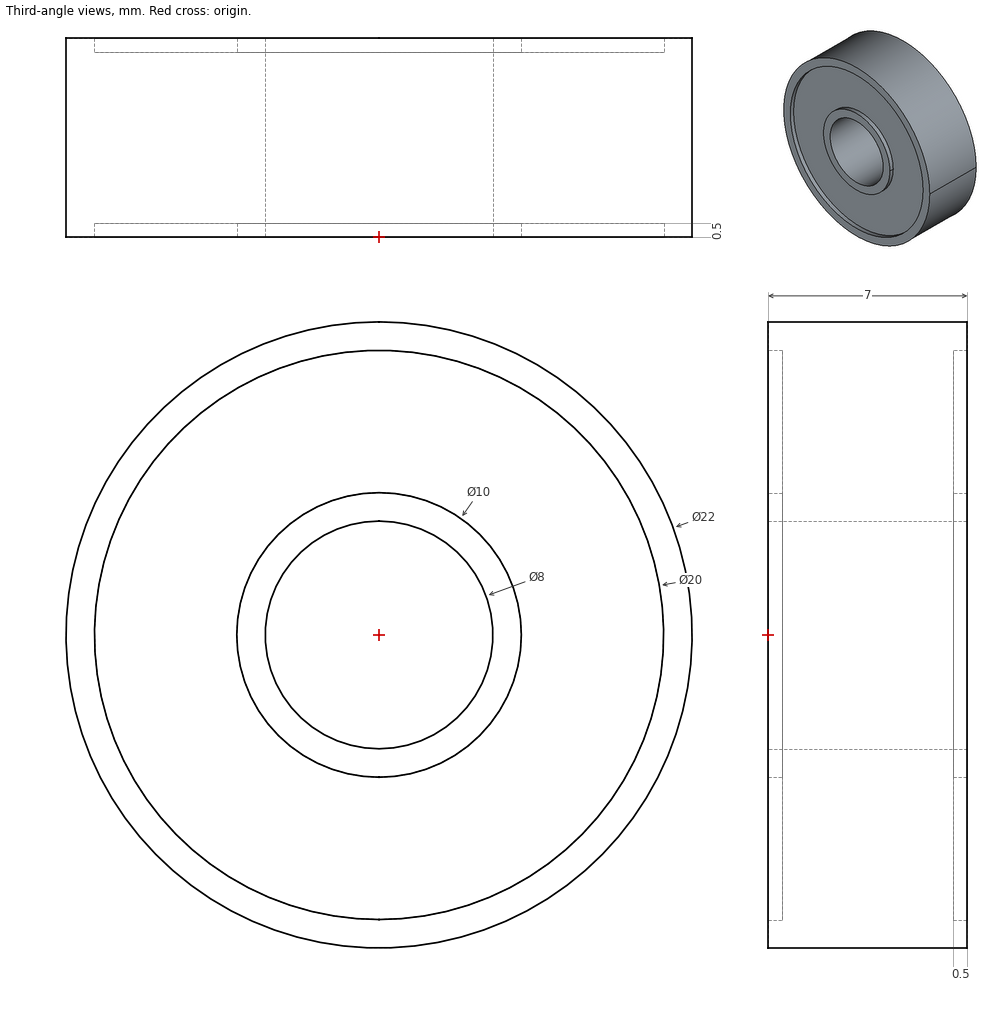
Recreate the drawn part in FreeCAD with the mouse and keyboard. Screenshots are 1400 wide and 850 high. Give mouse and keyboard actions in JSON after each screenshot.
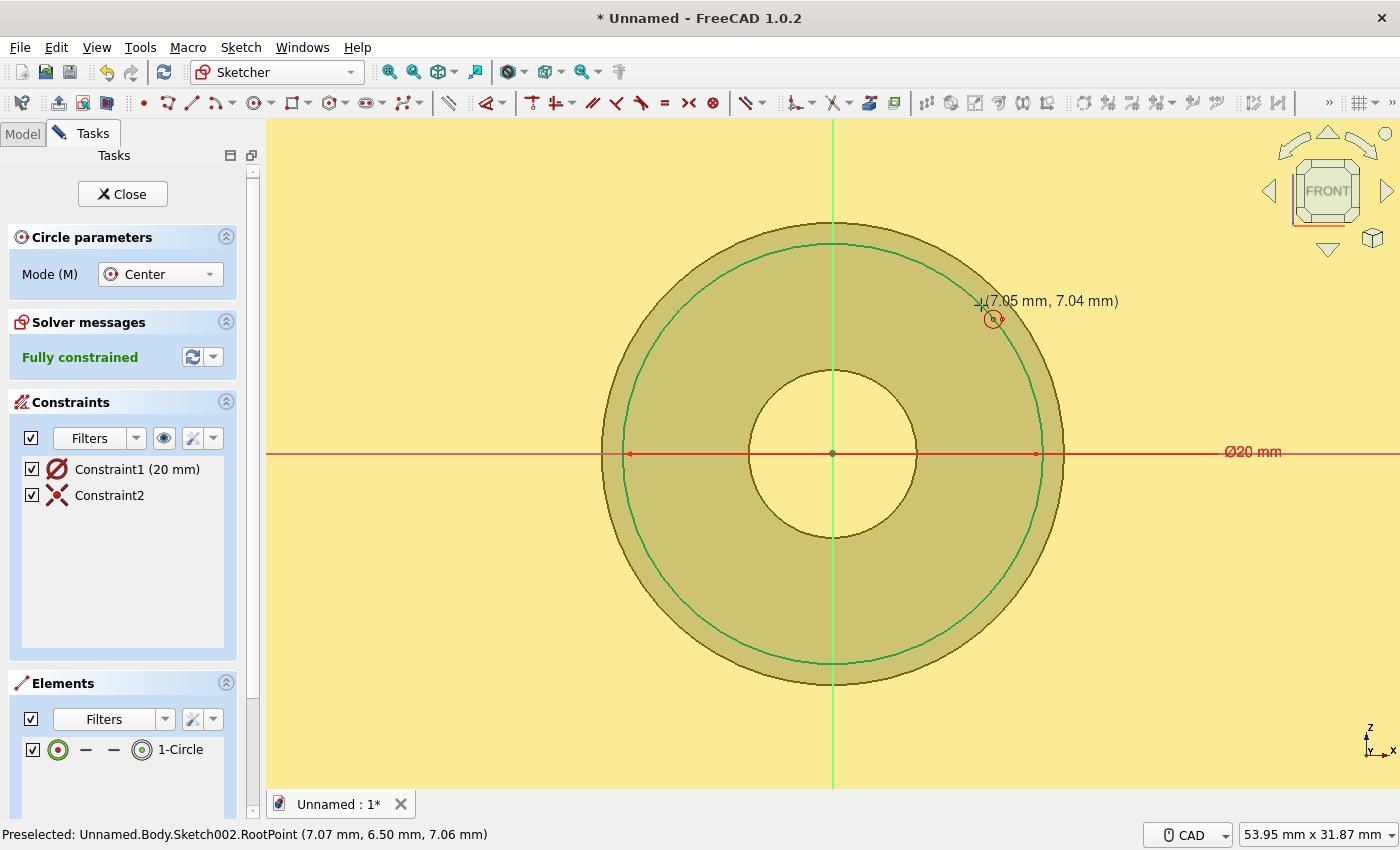
{"action": "left_click", "coordinate": [833, 454]}
{"action": "mouse_move", "coordinate": [907, 380]}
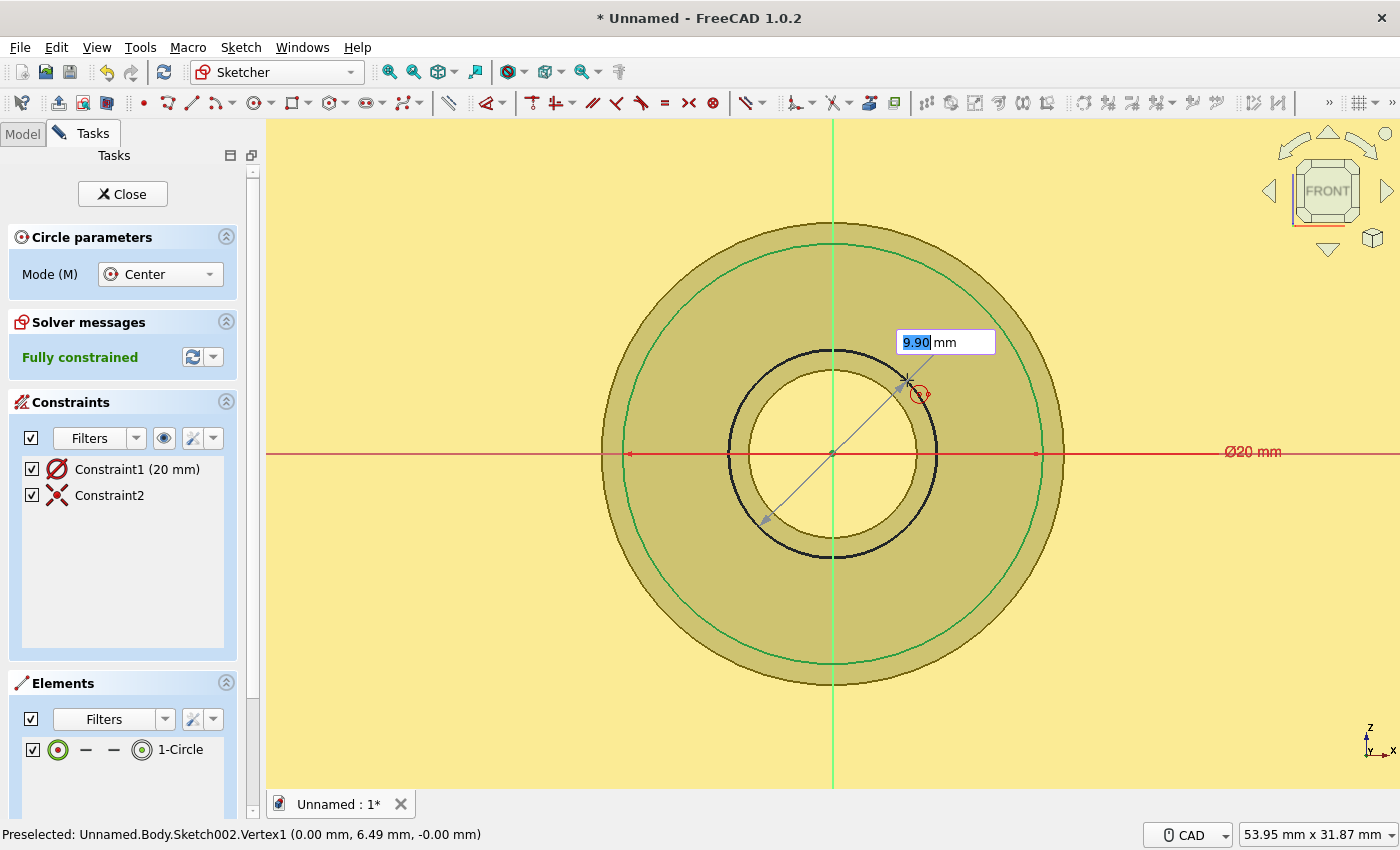
{"action": "type", "text": "10"}
{"action": "key", "text": "Return"}
{"action": "key", "text": "Escape"}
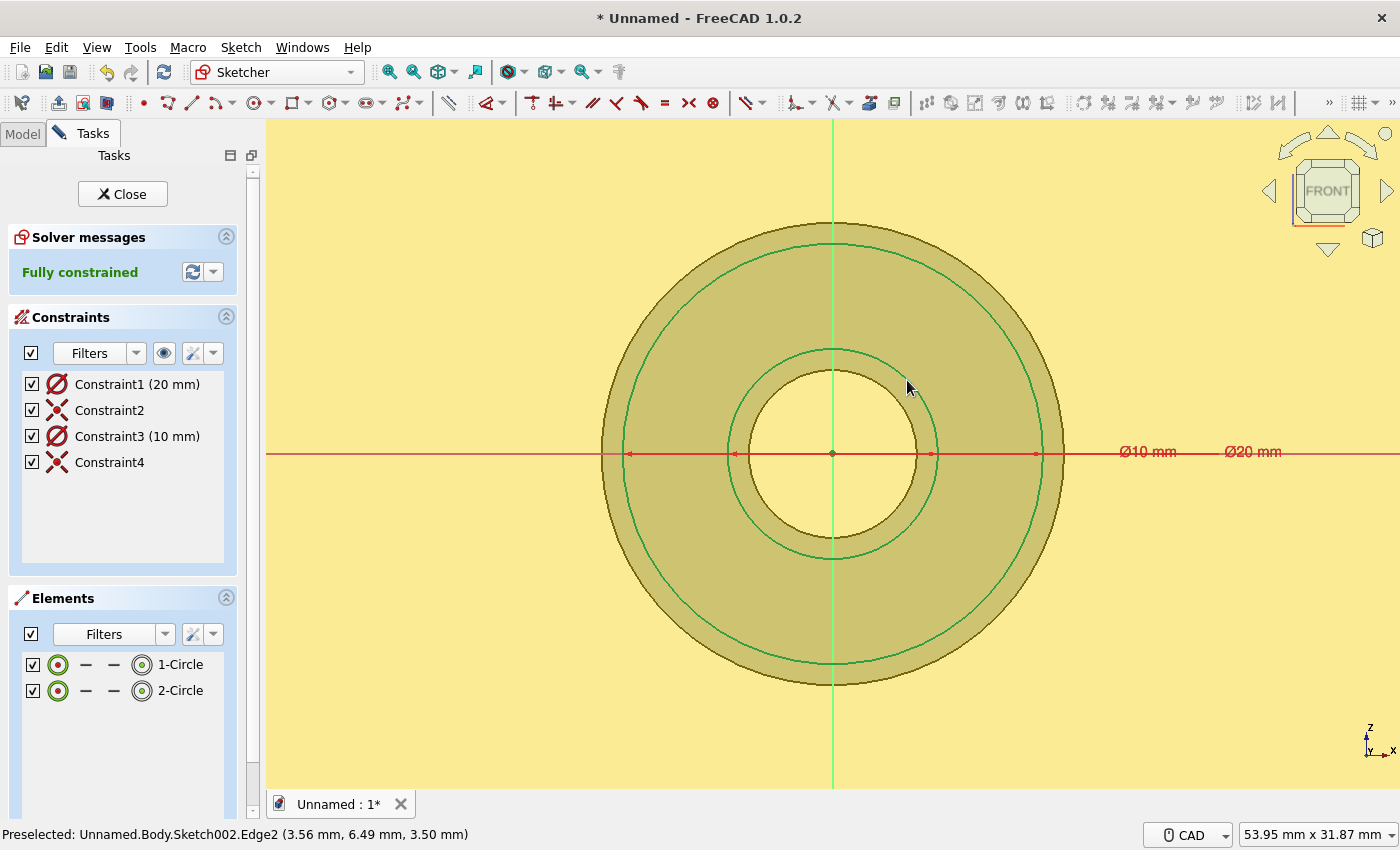
{"action": "left_click", "coordinate": [123, 194]}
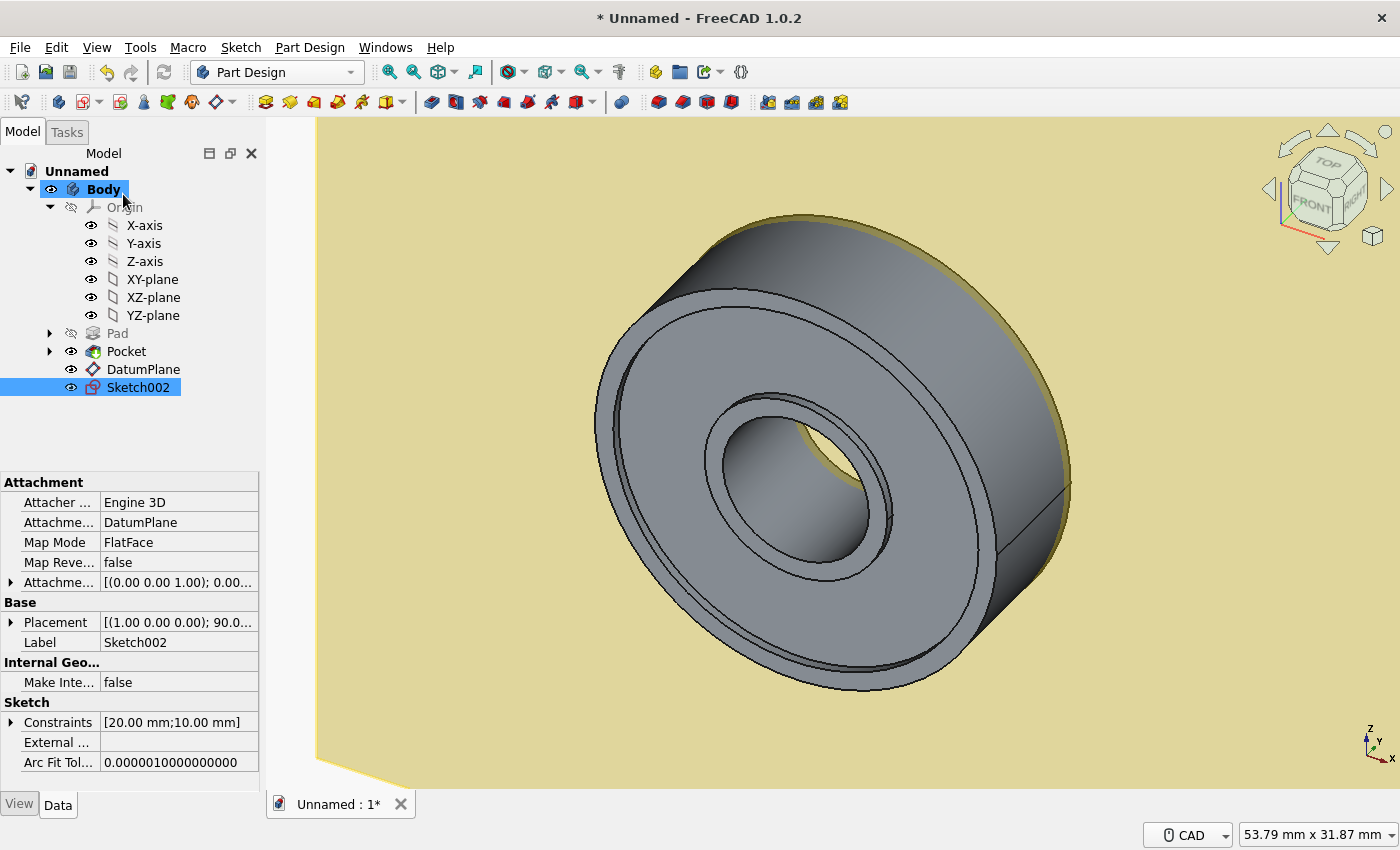
{"action": "left_click", "coordinate": [432, 102]}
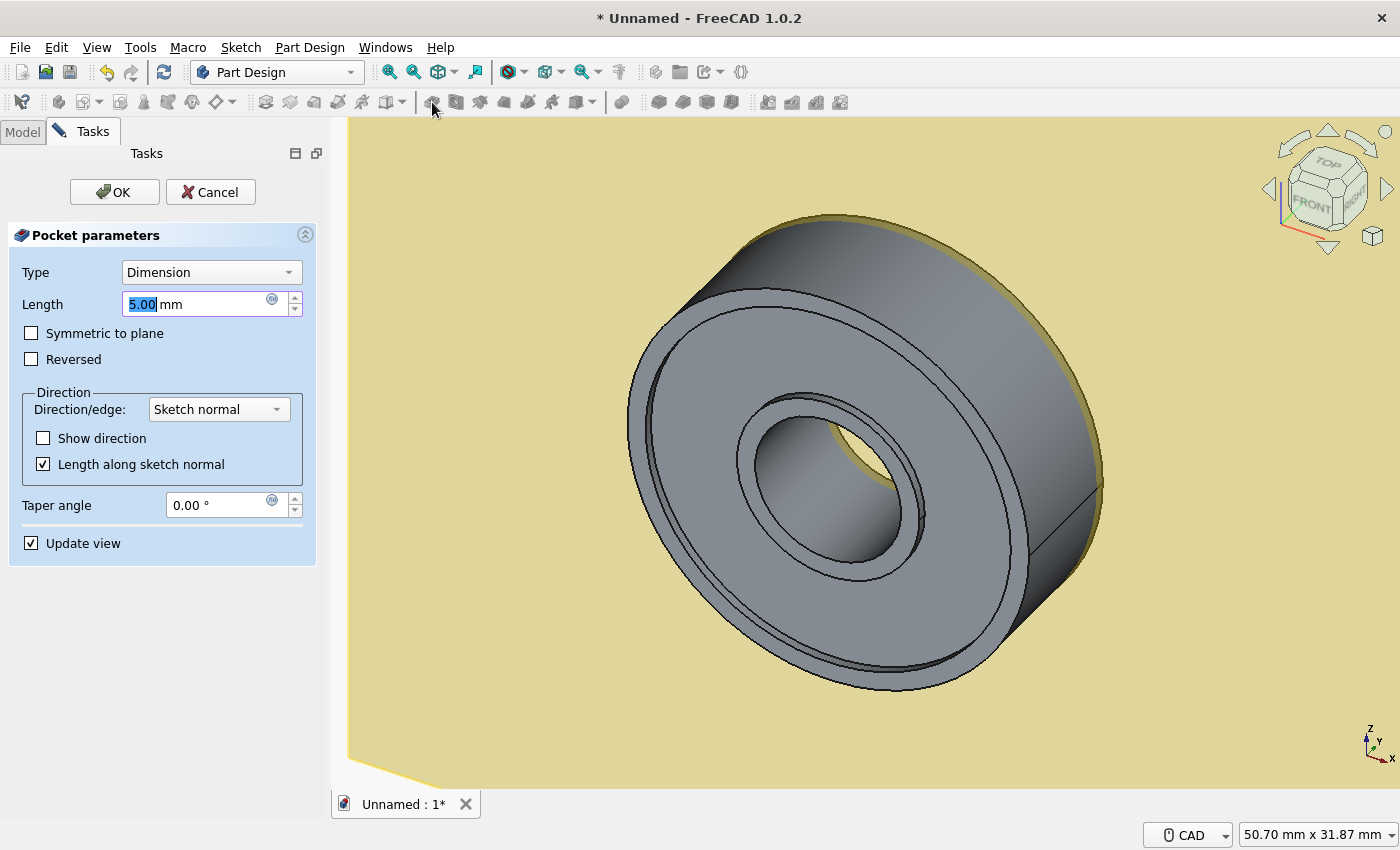
{"action": "type", "text": "0.5"}
{"action": "key", "text": "Tab"}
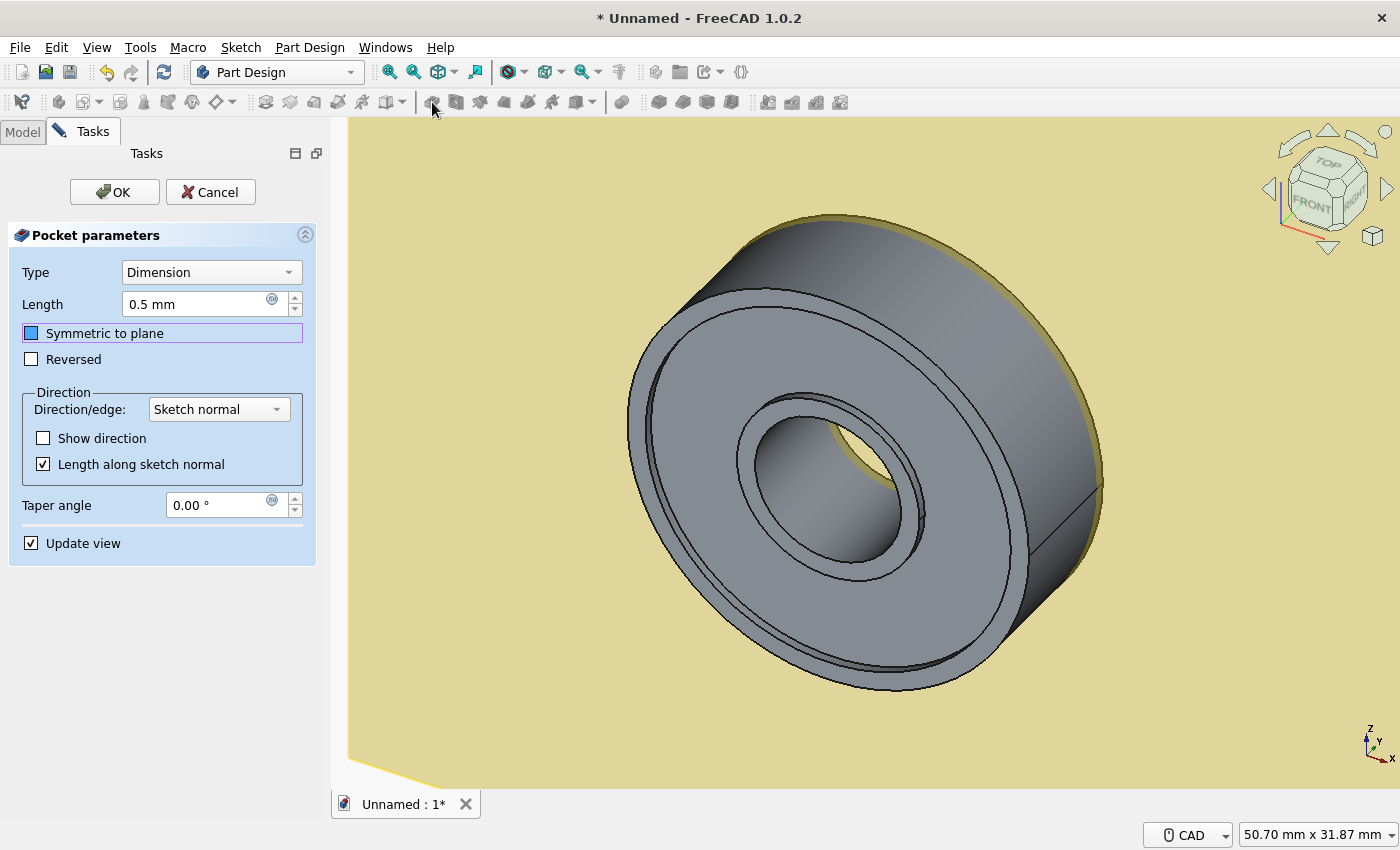
{"action": "left_click", "coordinate": [115, 192]}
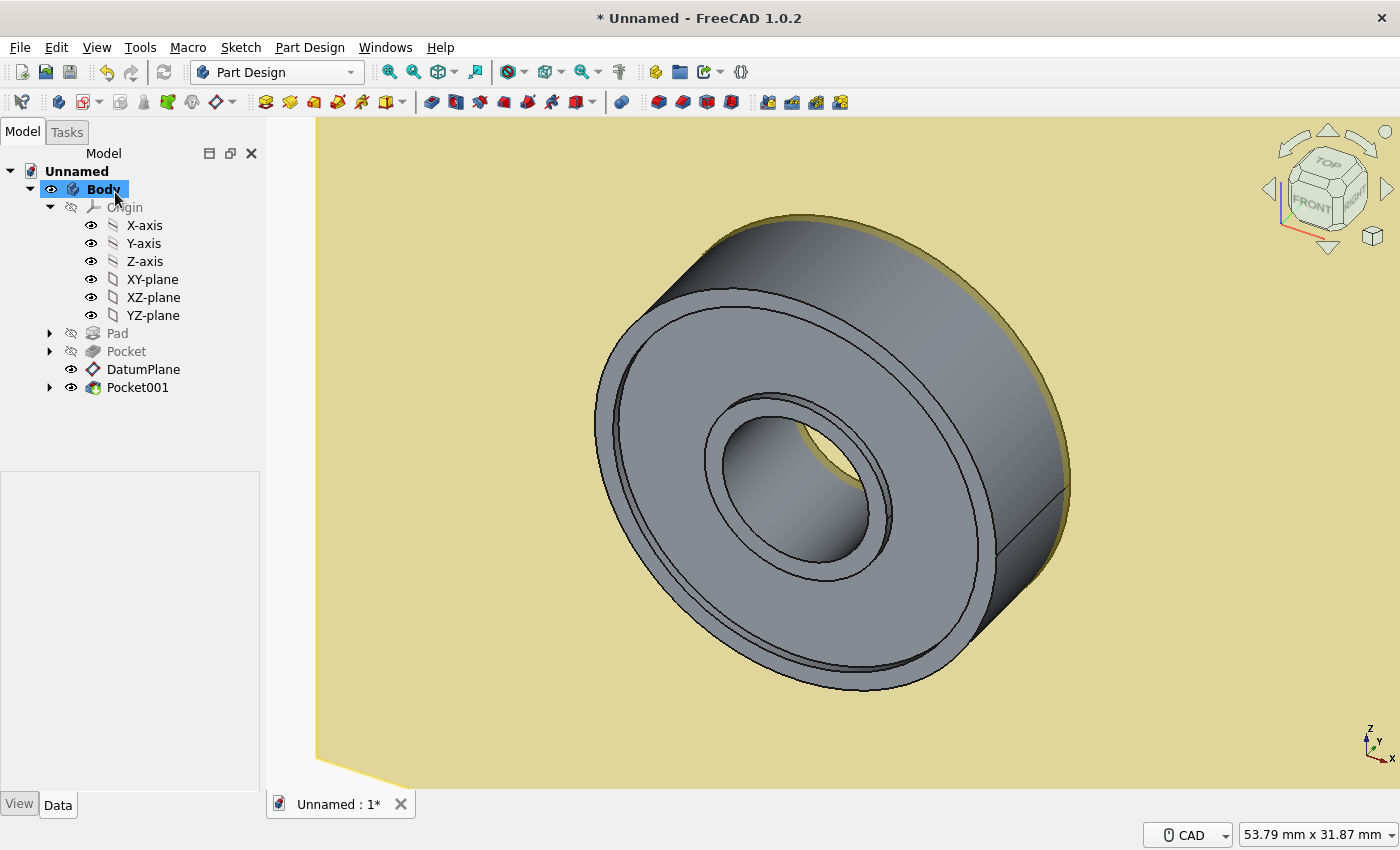
{"action": "left_click", "coordinate": [116, 369]}
{"action": "key", "text": "space"}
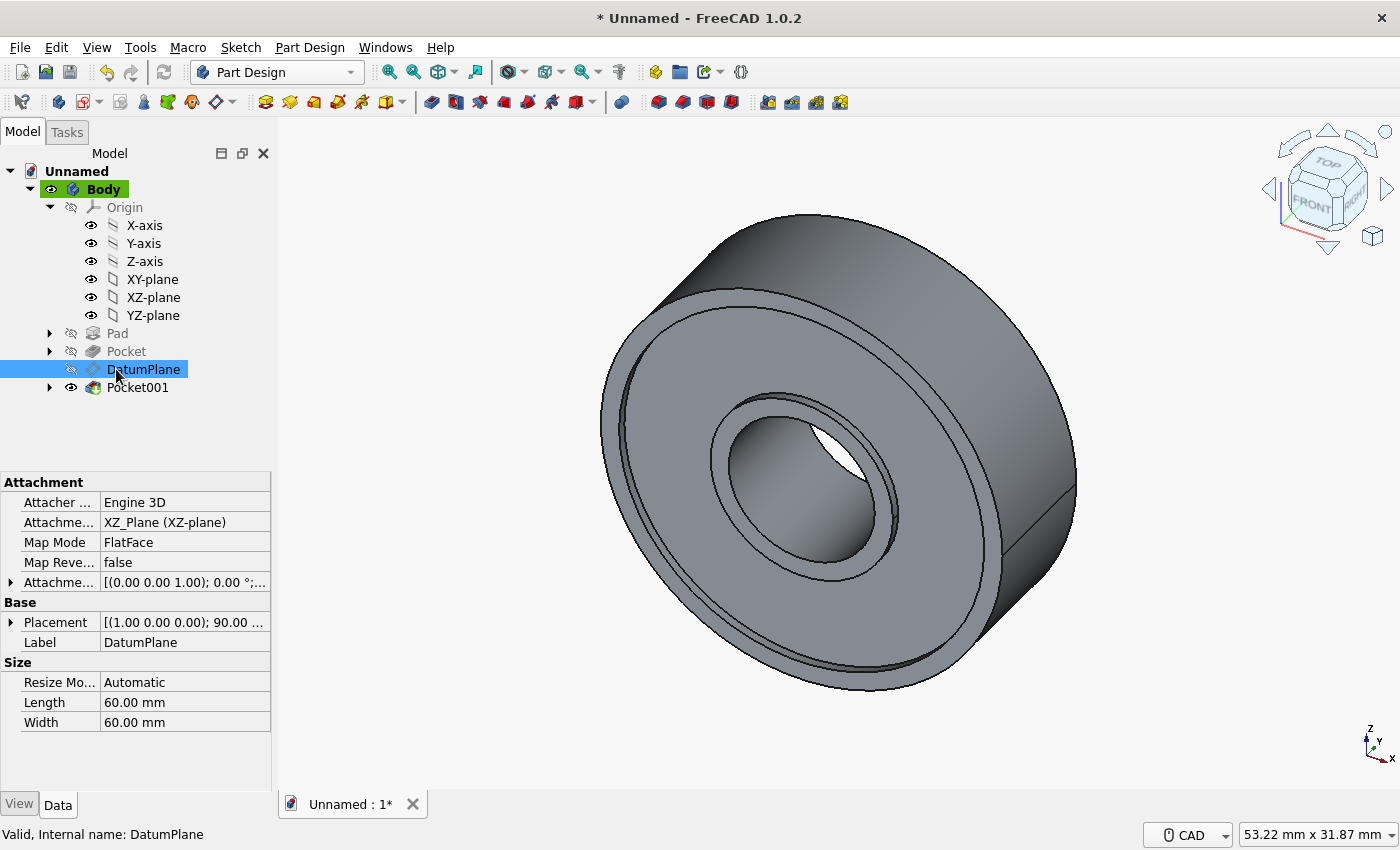
{"action": "key", "text": "0"}